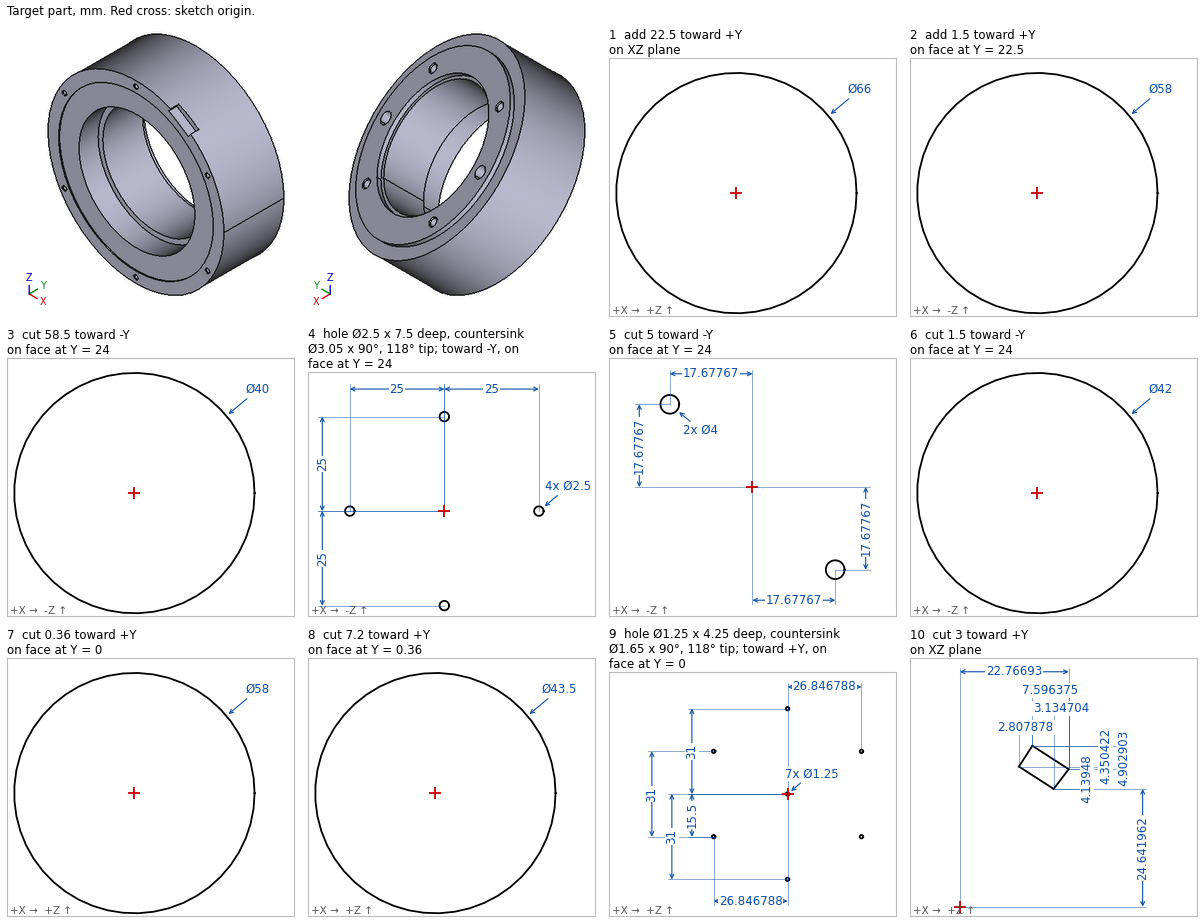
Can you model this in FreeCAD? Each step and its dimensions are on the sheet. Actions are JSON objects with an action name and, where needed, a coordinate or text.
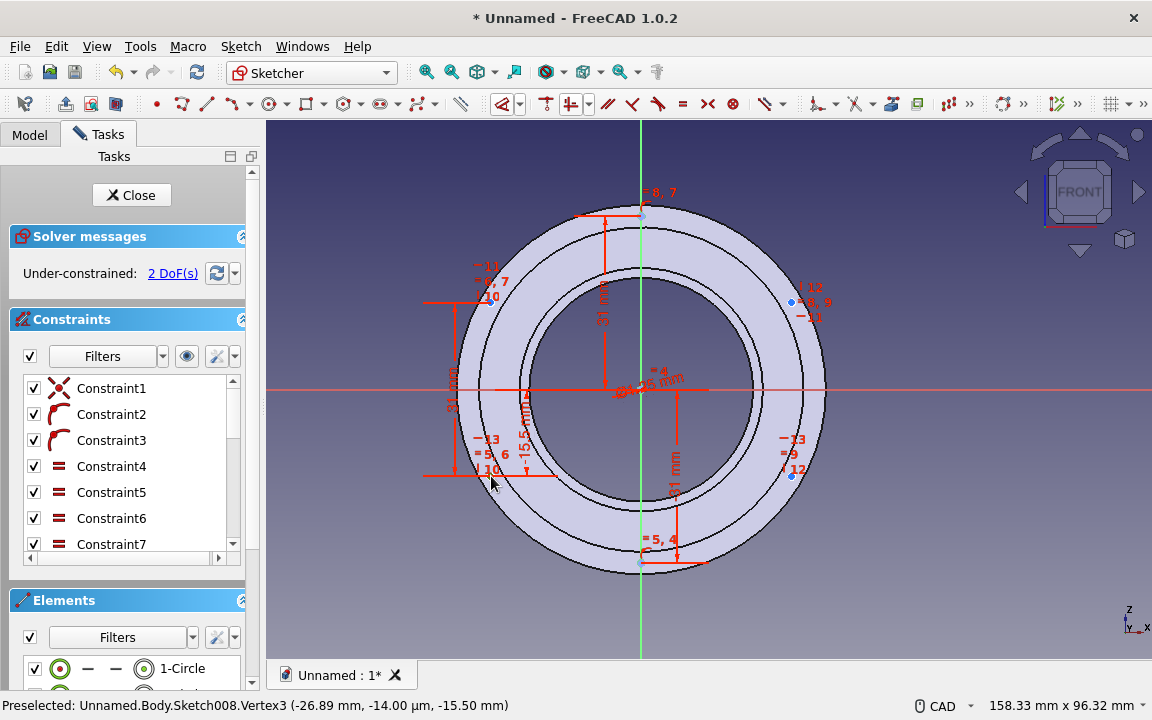
{"action": "left_click", "coordinate": [520, 104]}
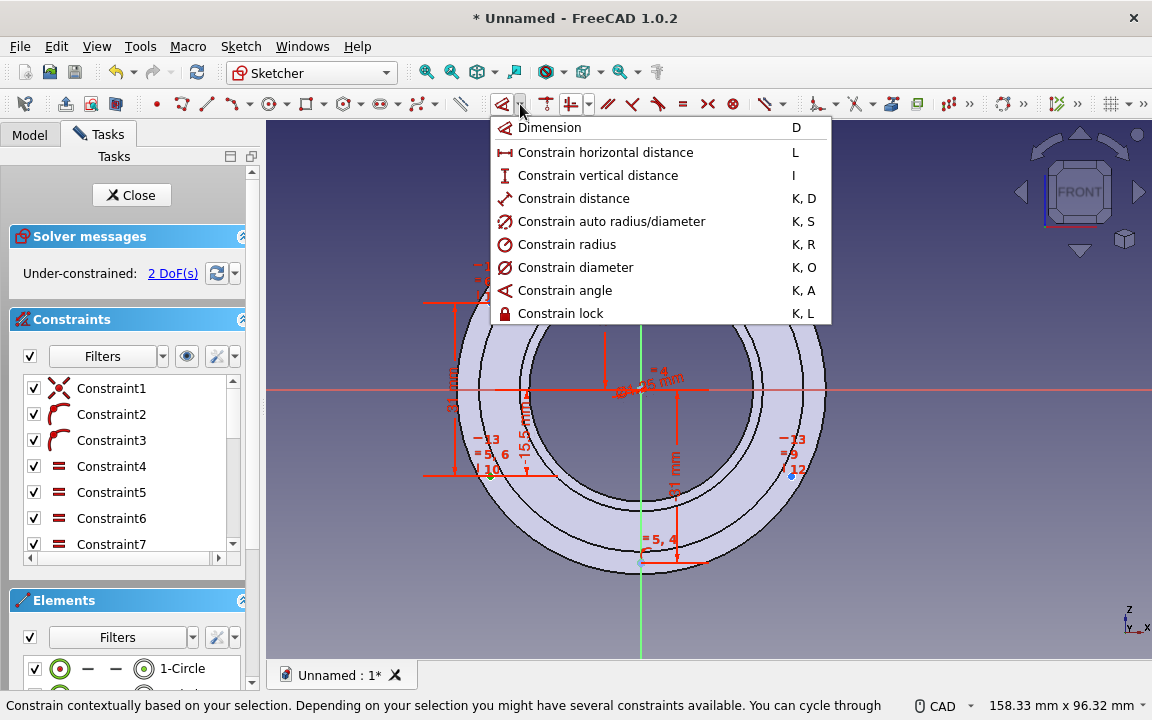
{"action": "left_click", "coordinate": [661, 152]}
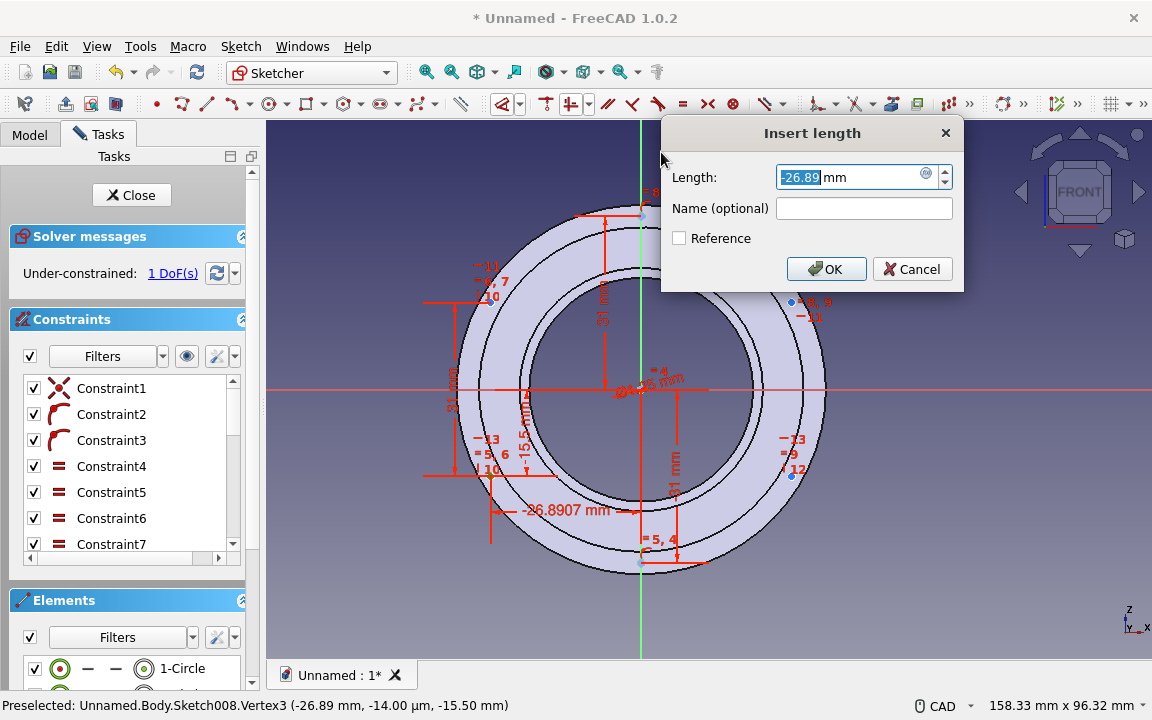
{"action": "type", "text": "-26.846788"}
{"action": "key", "text": "Return"}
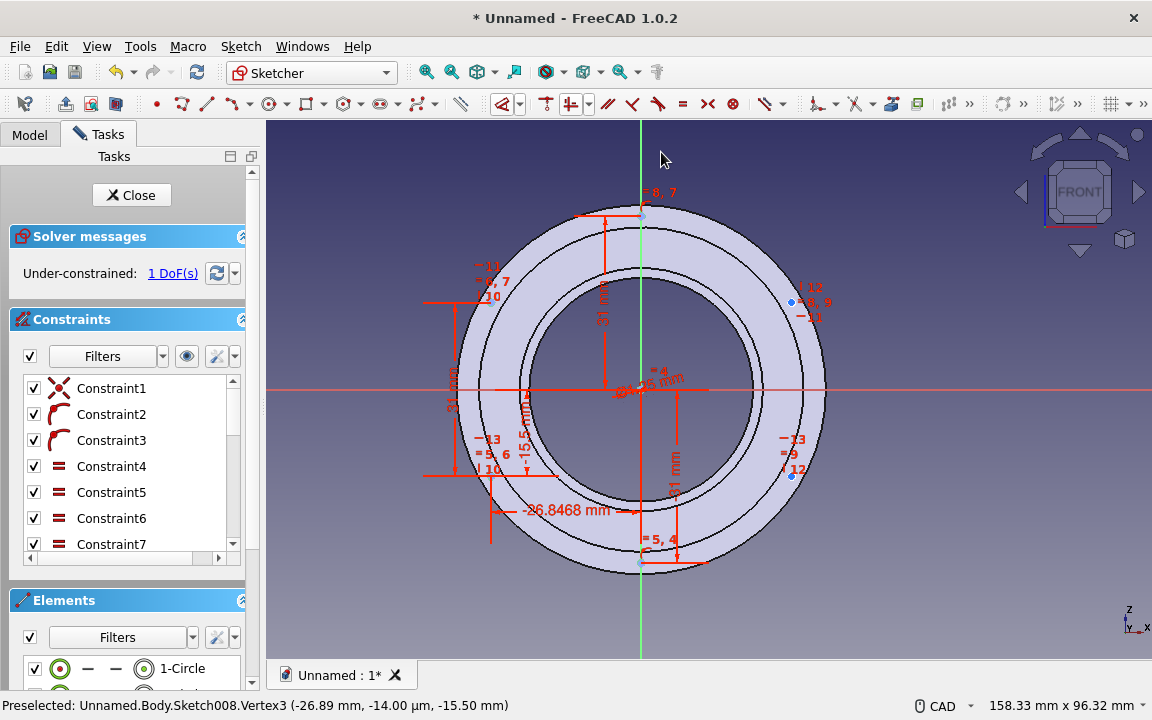
{"action": "left_click", "coordinate": [792, 303]}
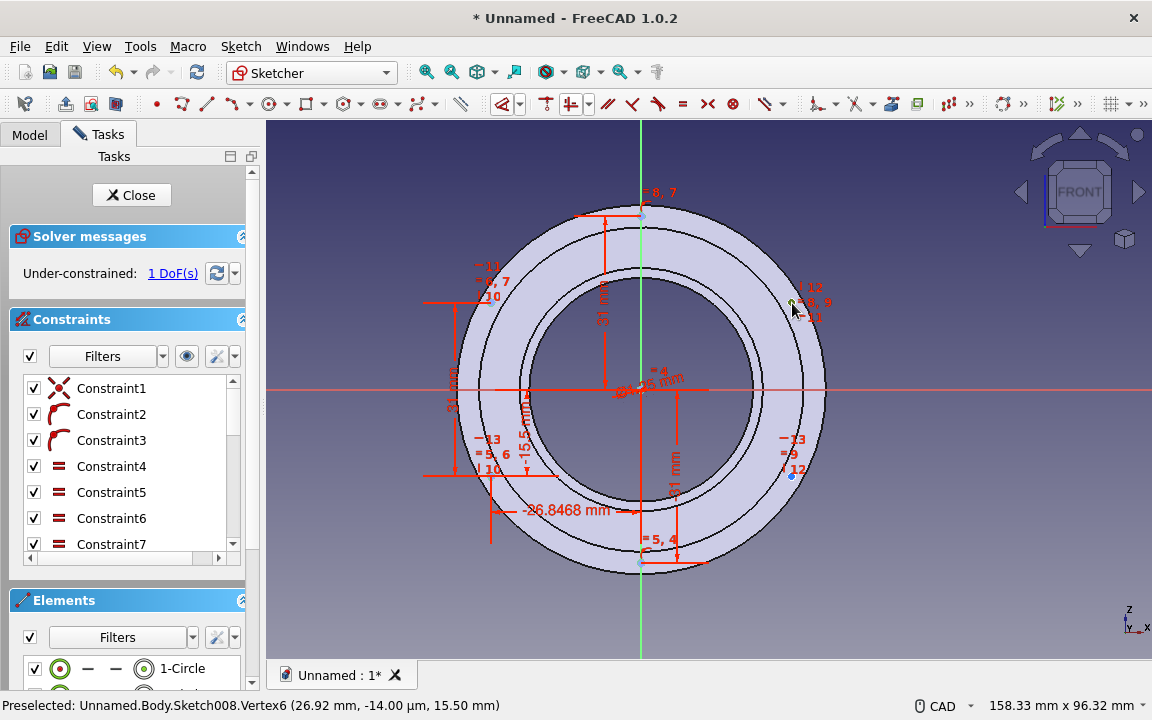
{"action": "left_click", "coordinate": [520, 104]}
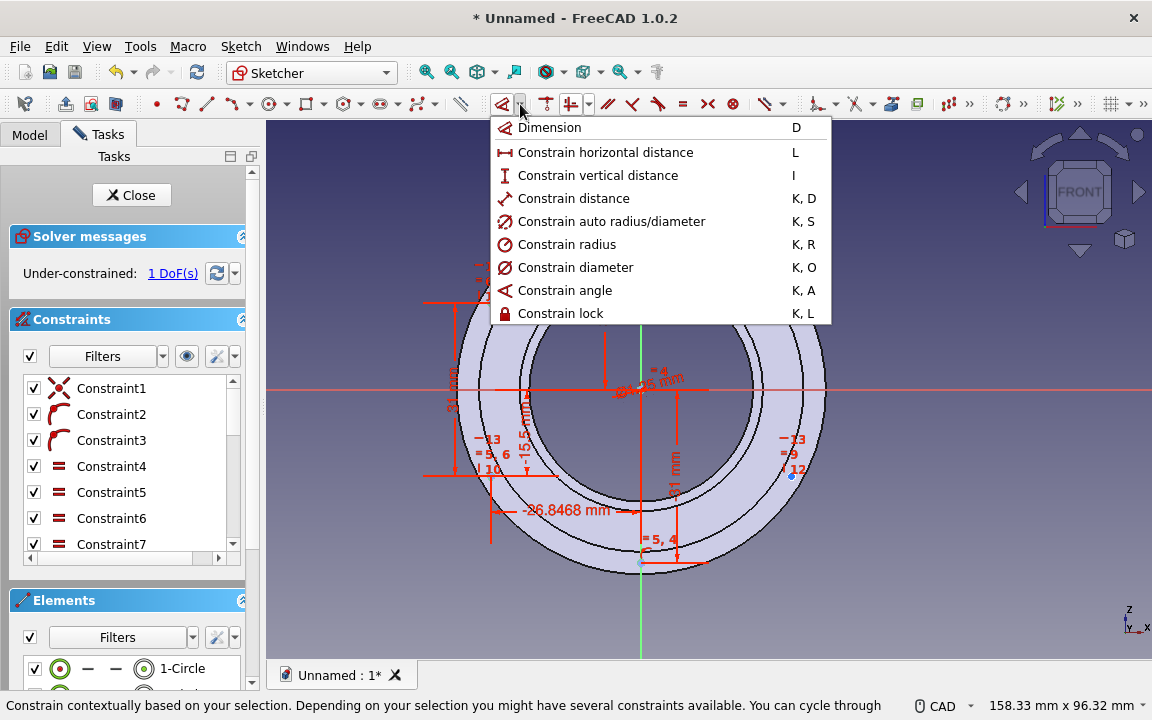
{"action": "left_click", "coordinate": [661, 152]}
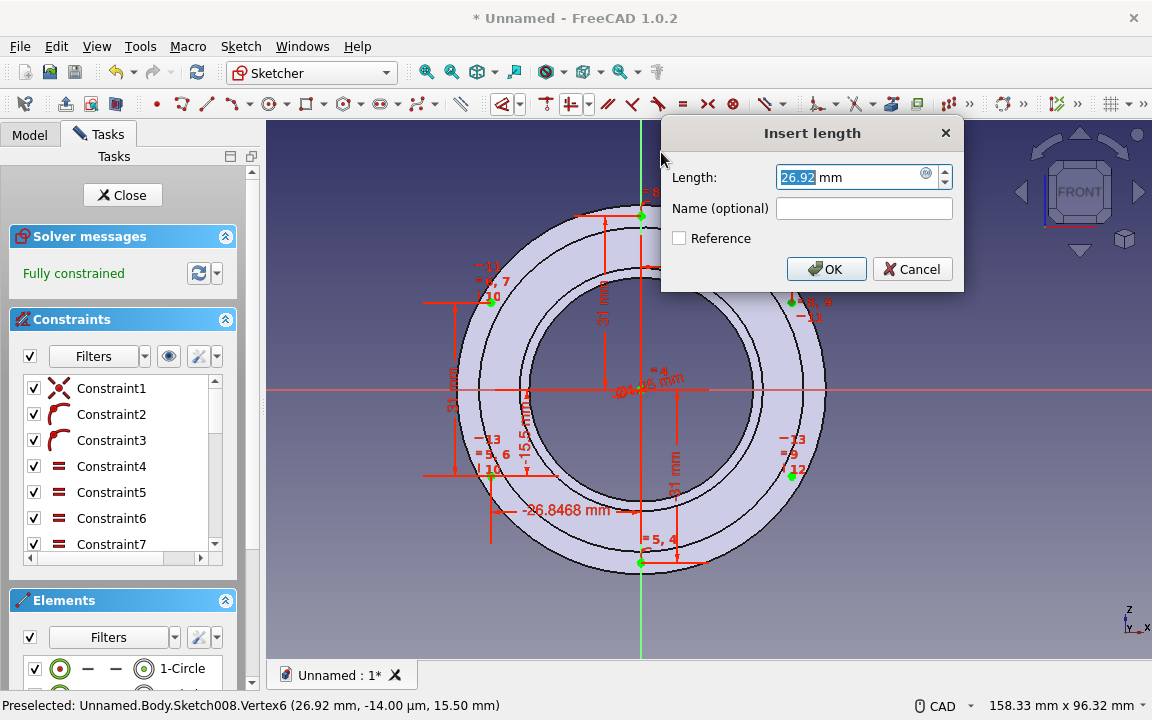
{"action": "type", "text": "26.846788"}
{"action": "key", "text": "Return"}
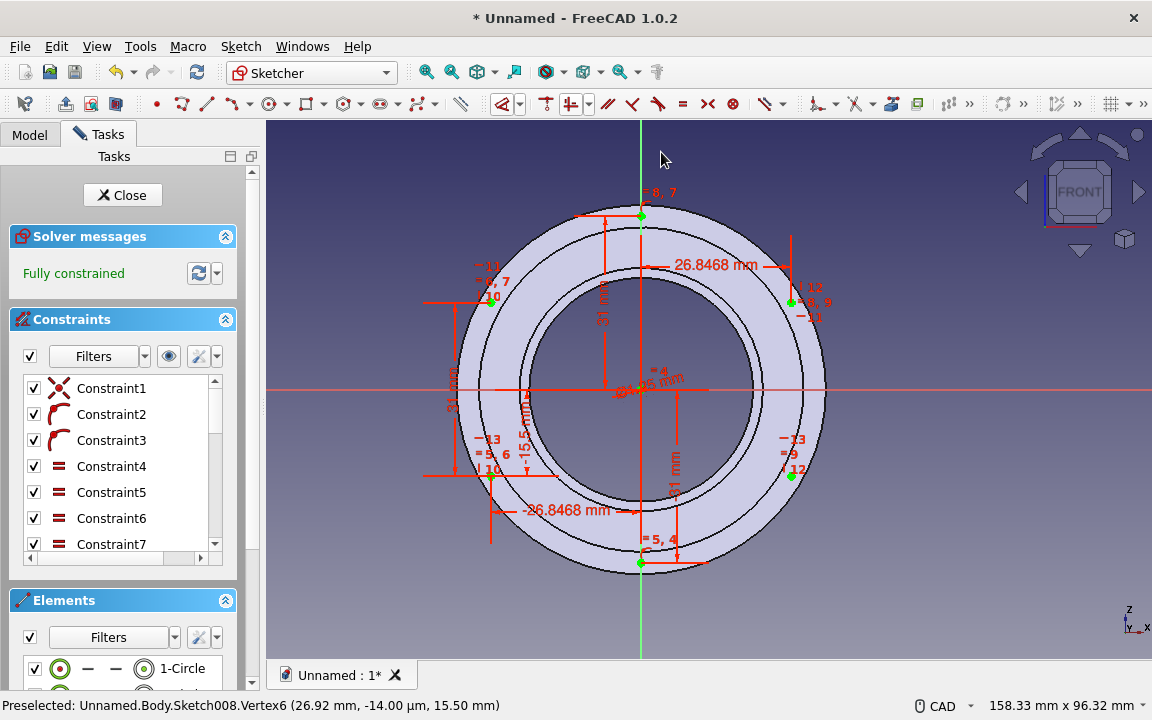
{"action": "left_click", "coordinate": [123, 195]}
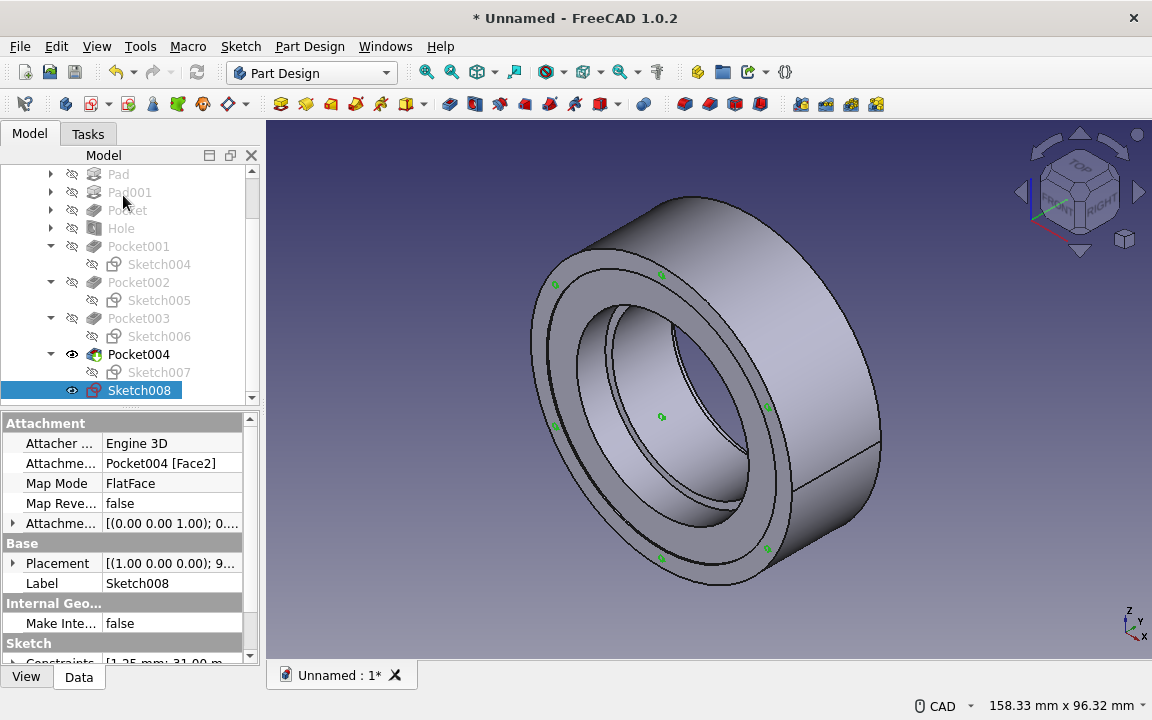
{"action": "left_click", "coordinate": [475, 104]}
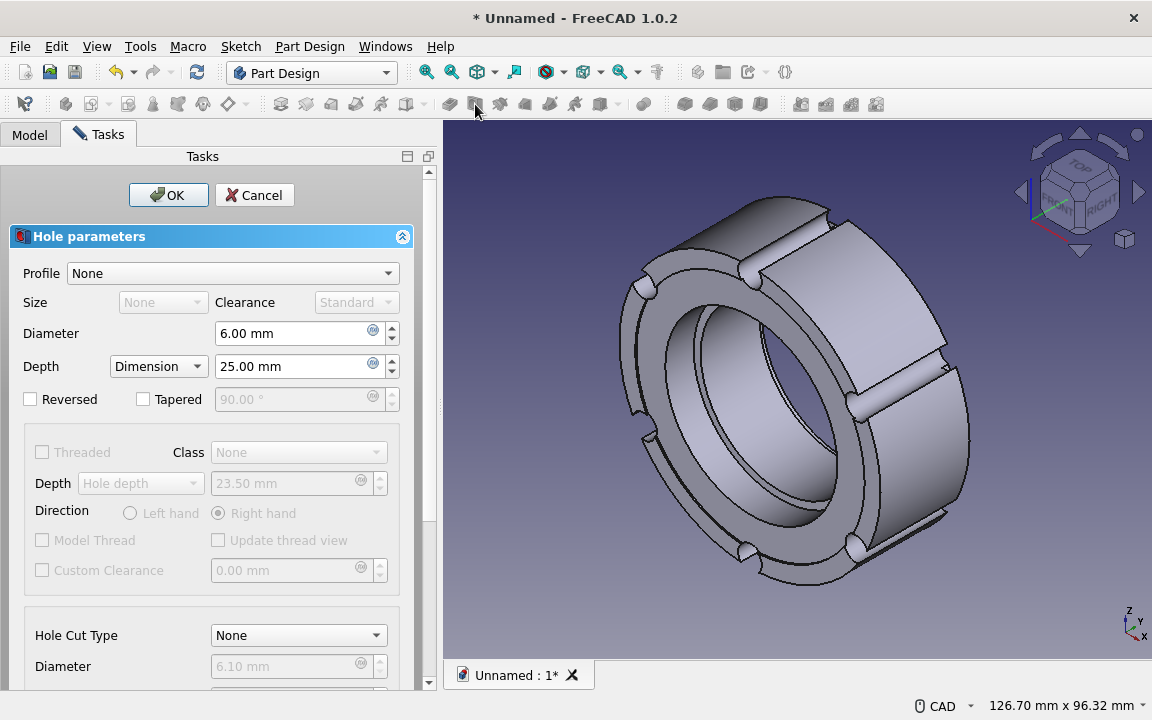
{"action": "triple_click", "coordinate": [300, 334]}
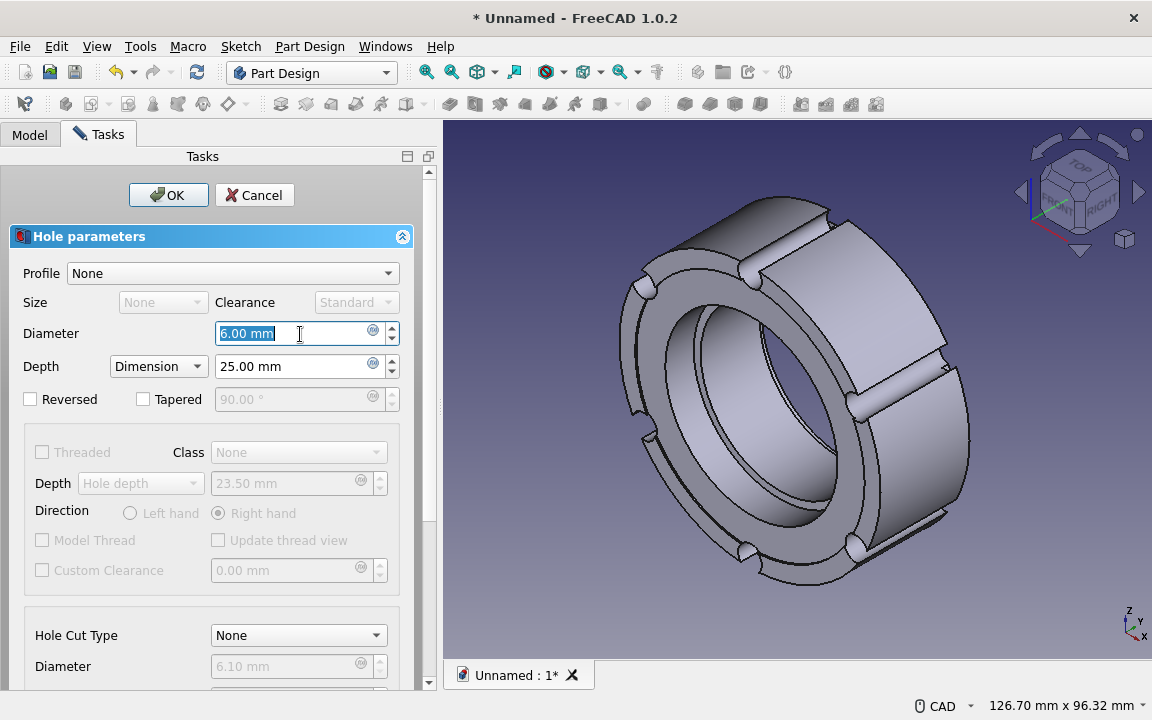
{"action": "type", "text": "1.25"}
{"action": "key", "text": "Tab"}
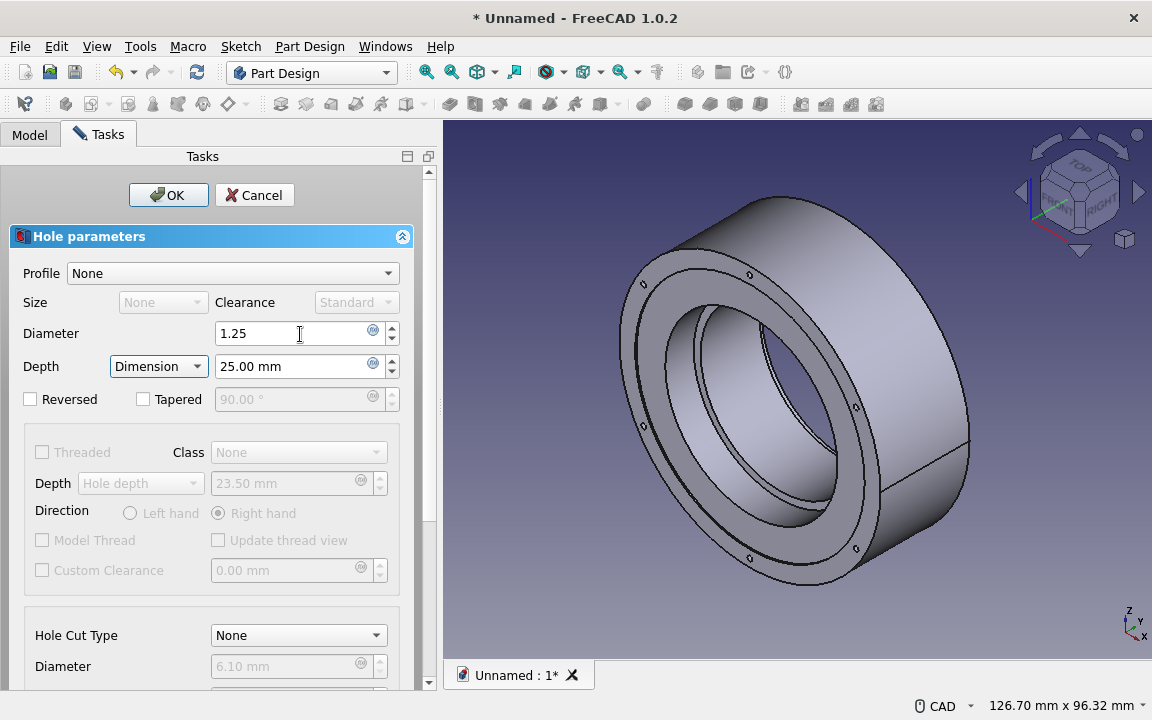
{"action": "triple_click", "coordinate": [300, 366]}